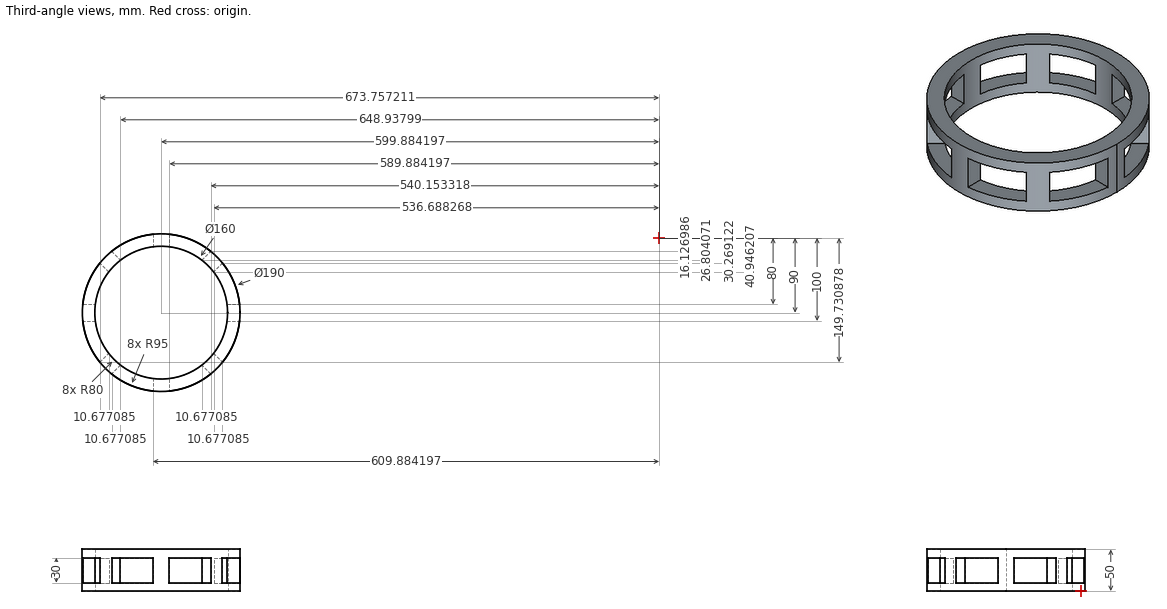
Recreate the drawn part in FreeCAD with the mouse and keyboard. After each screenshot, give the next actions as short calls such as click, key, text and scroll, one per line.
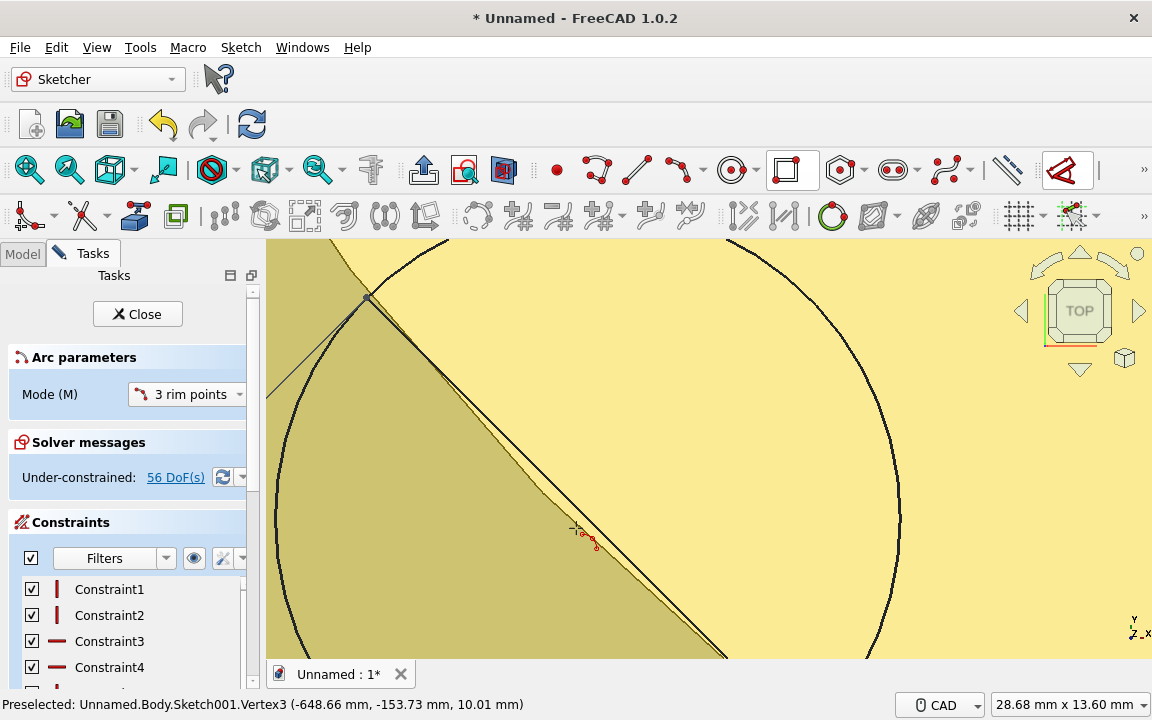
click(568, 518)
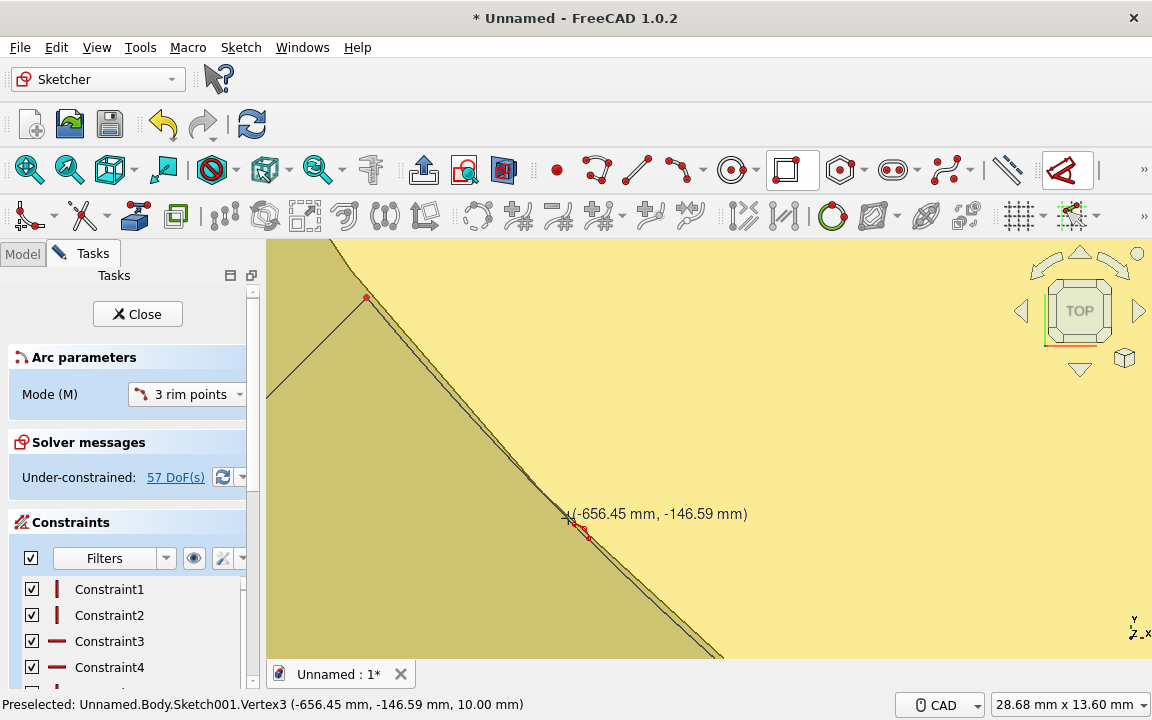
scroll(553, 537, down, 15)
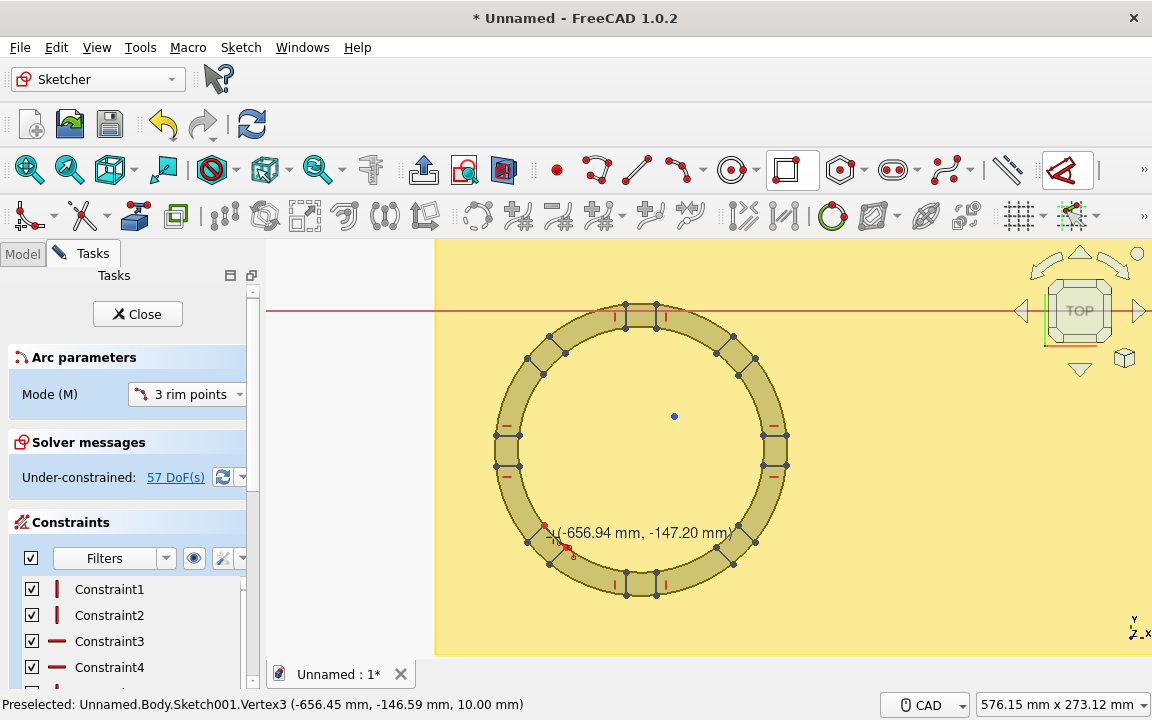
scroll(549, 563, up, 2)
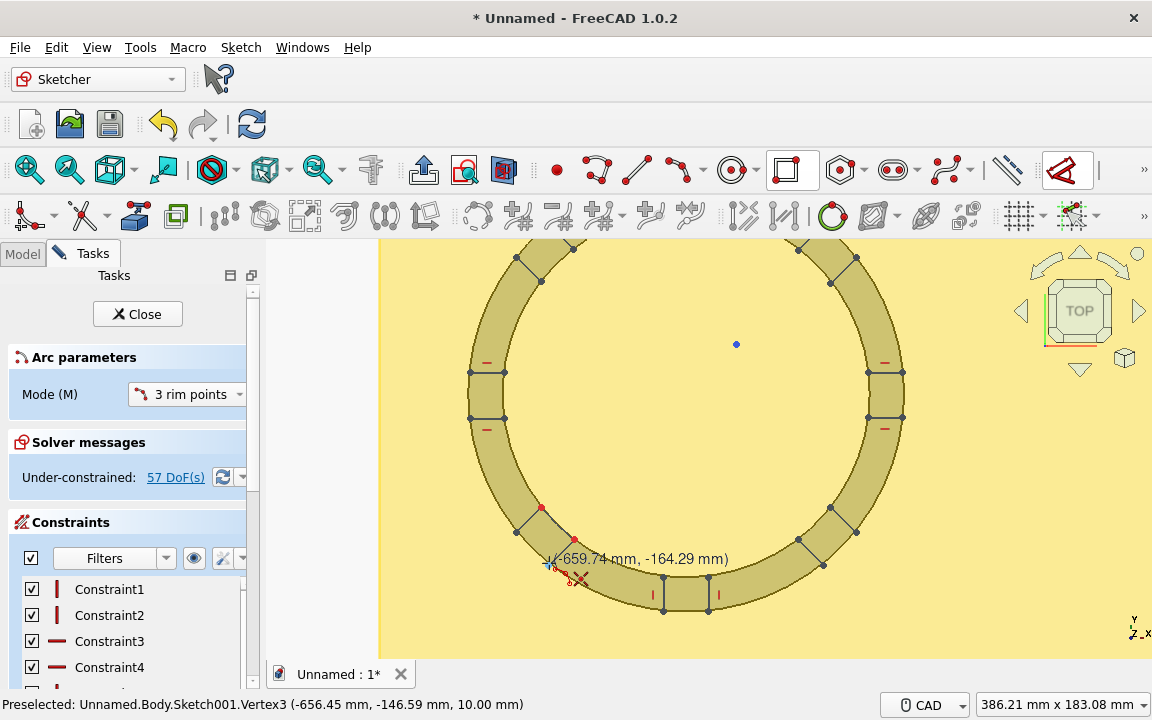
click(549, 565)
click(664, 611)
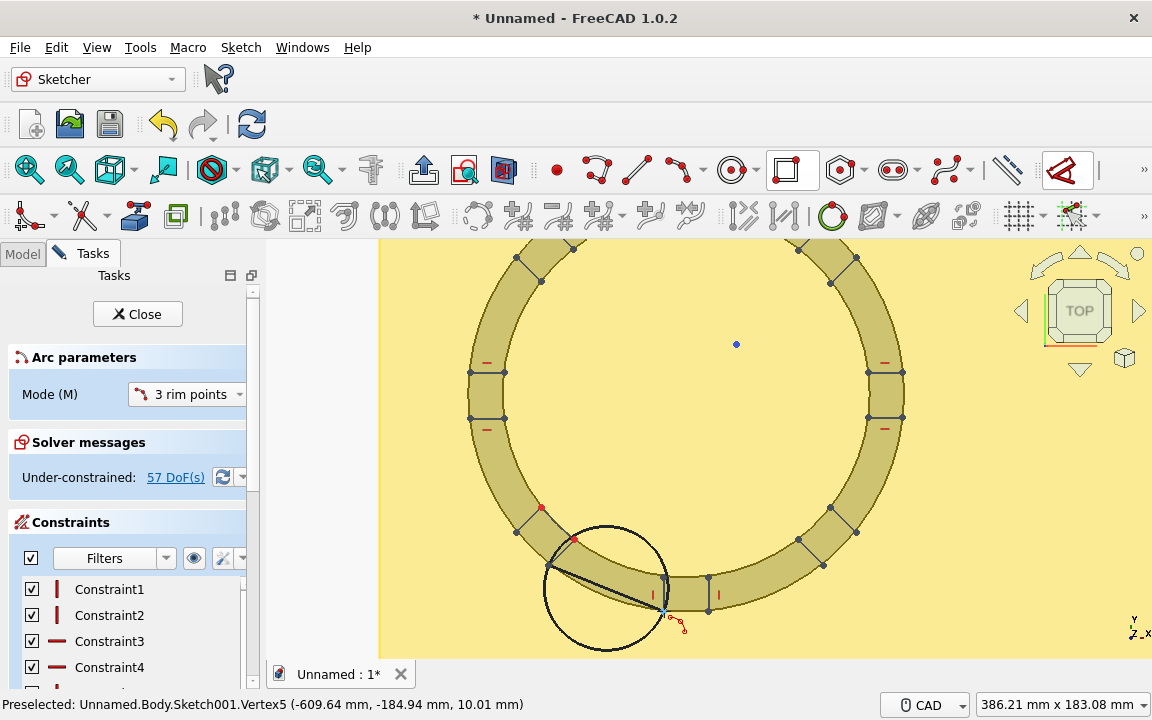
scroll(603, 595, up, 3)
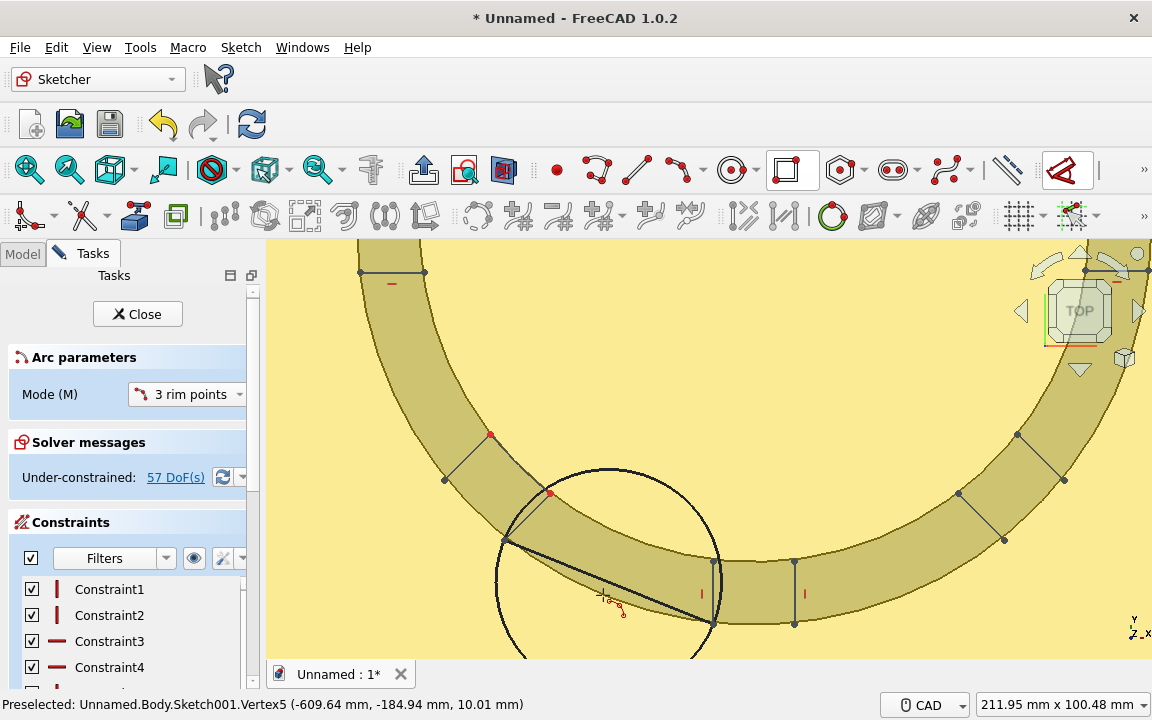
click(602, 594)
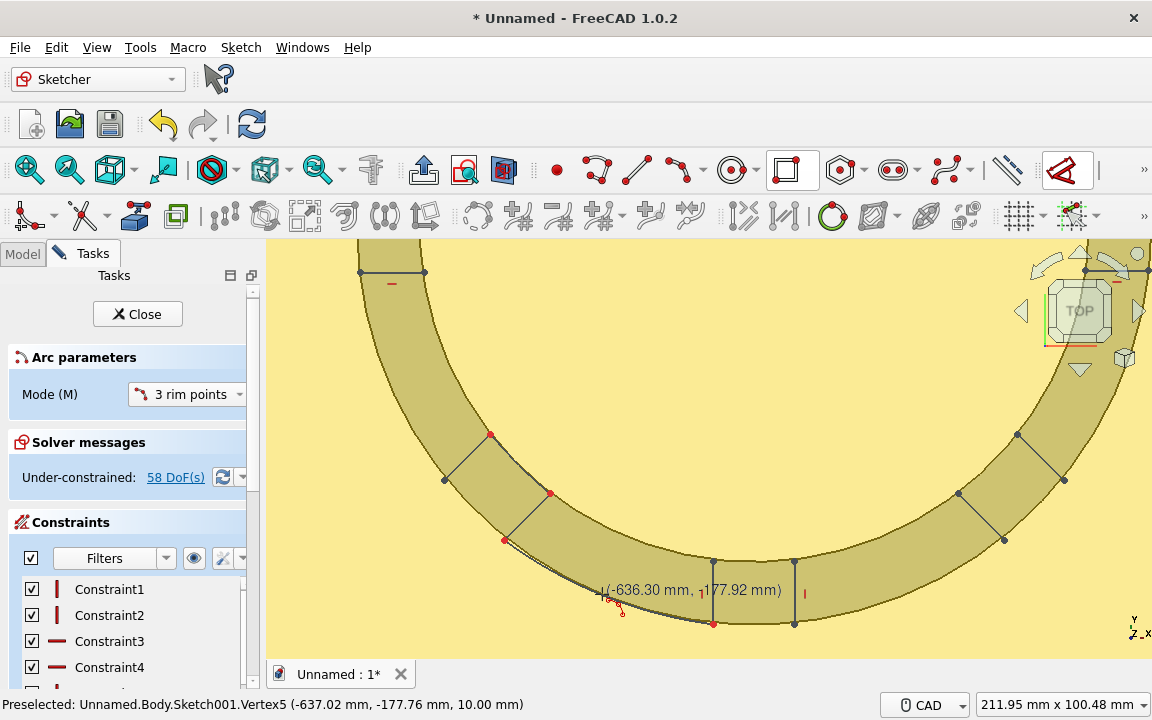
click(713, 562)
click(795, 562)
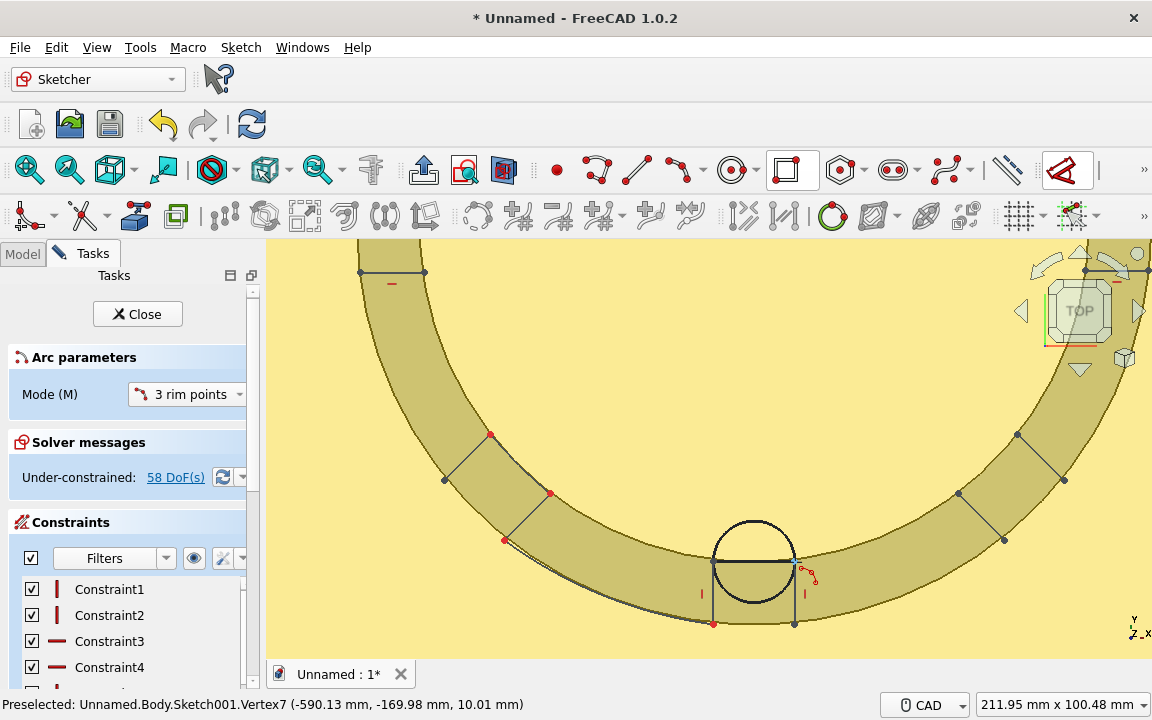
scroll(754, 562, up, 10)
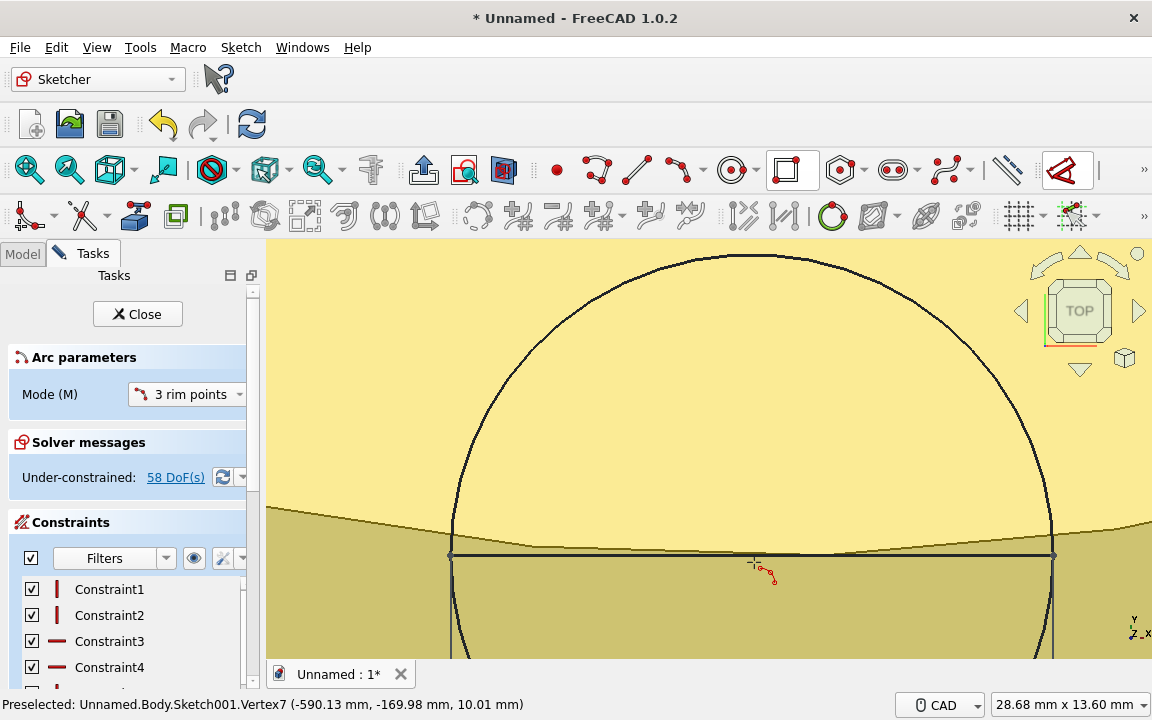
click(752, 556)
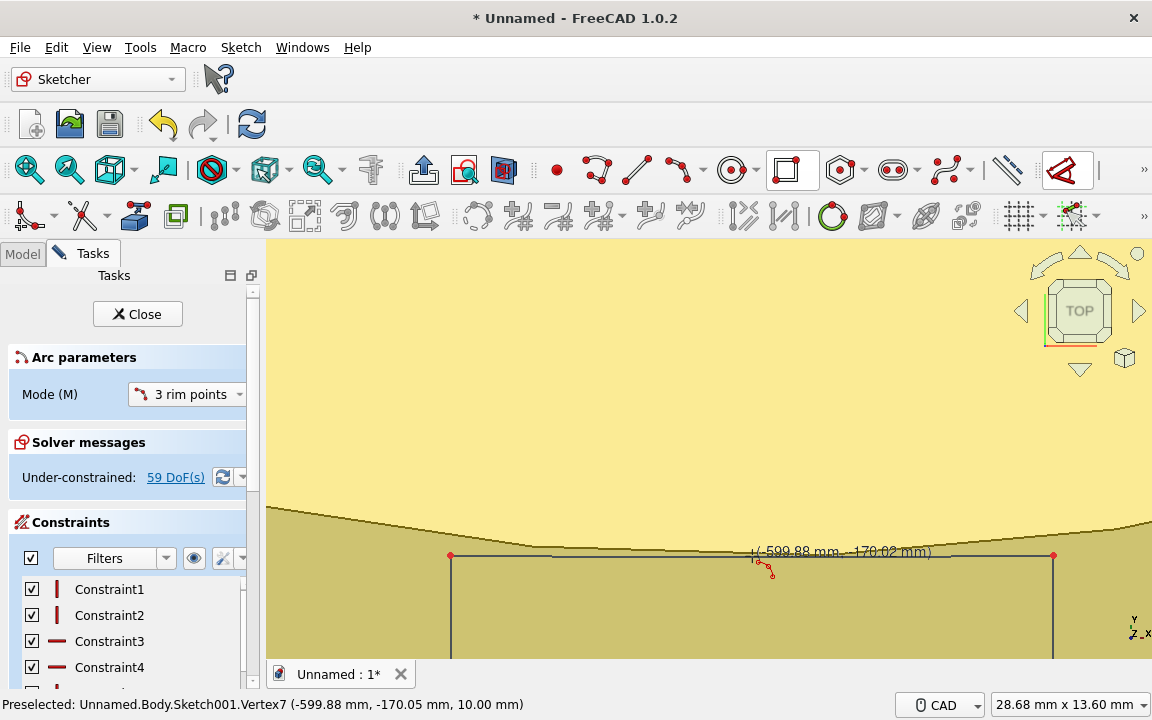
scroll(635, 573, down, 15)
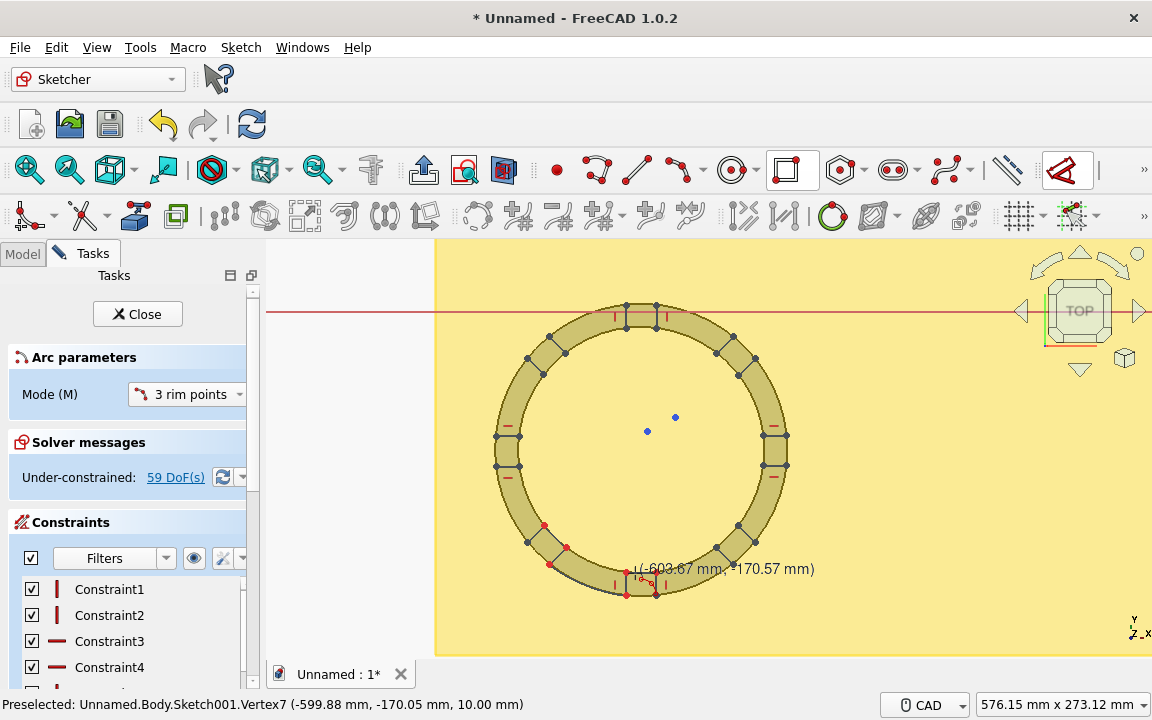
scroll(657, 595, up, 2)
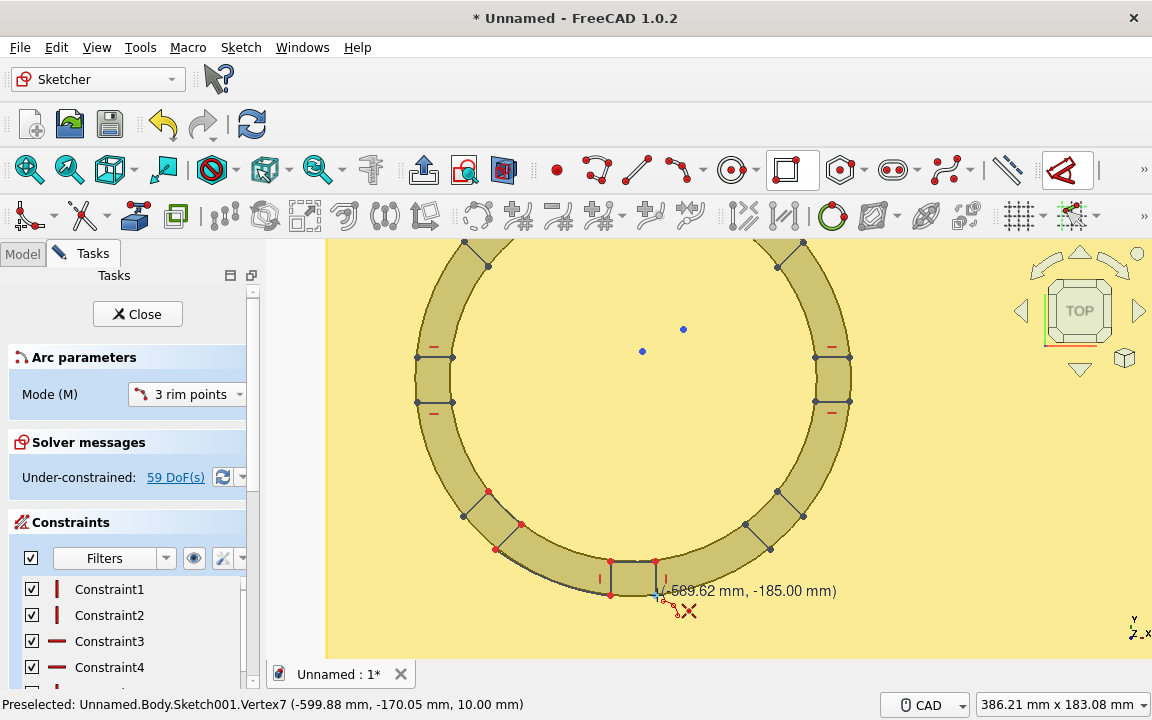
click(656, 596)
click(770, 550)